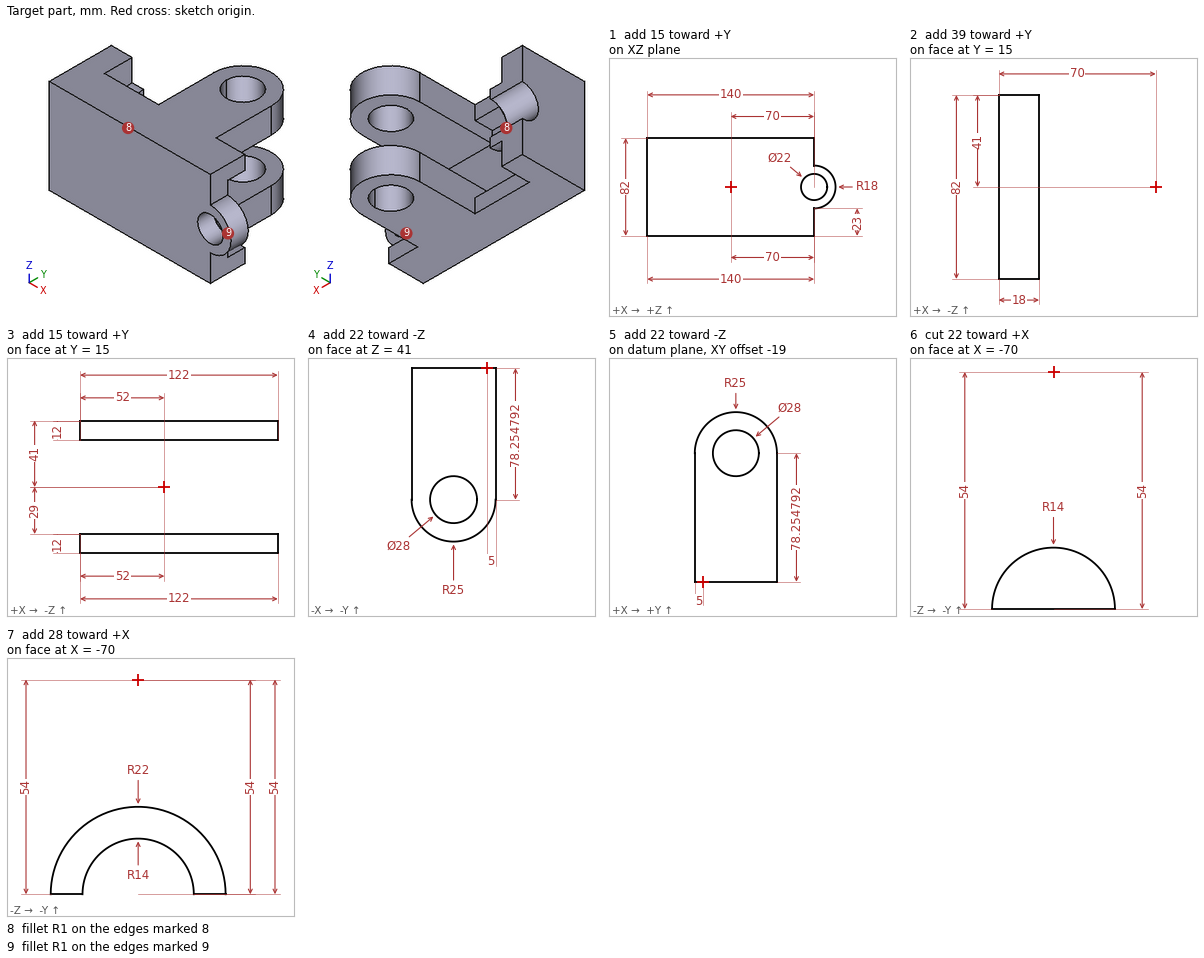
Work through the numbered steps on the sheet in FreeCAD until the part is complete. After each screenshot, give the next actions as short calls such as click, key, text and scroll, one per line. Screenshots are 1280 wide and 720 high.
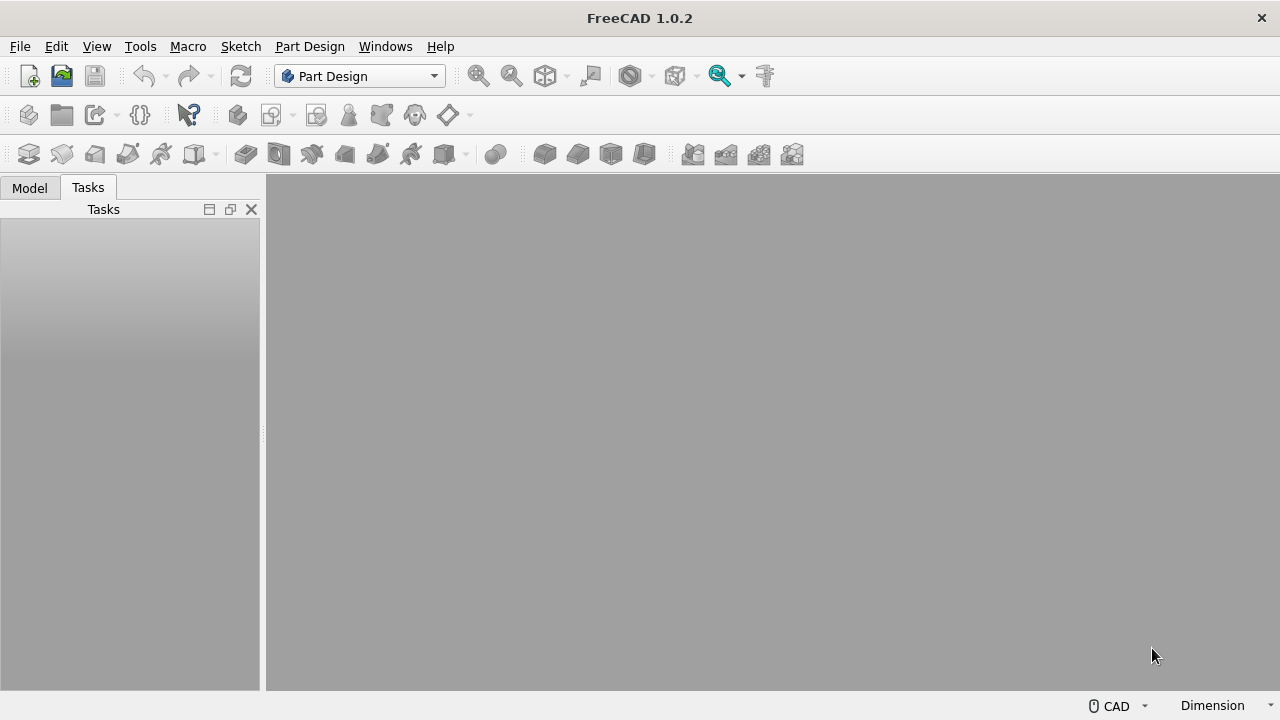
click(29, 76)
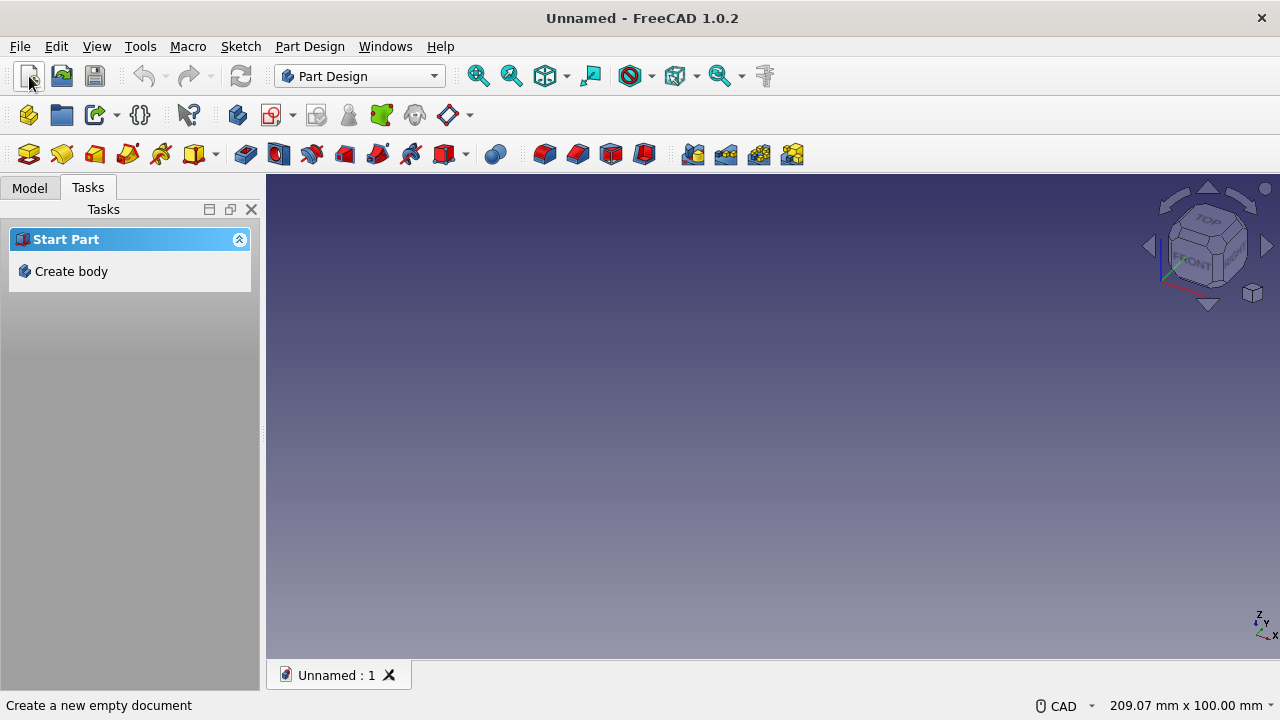
click(270, 116)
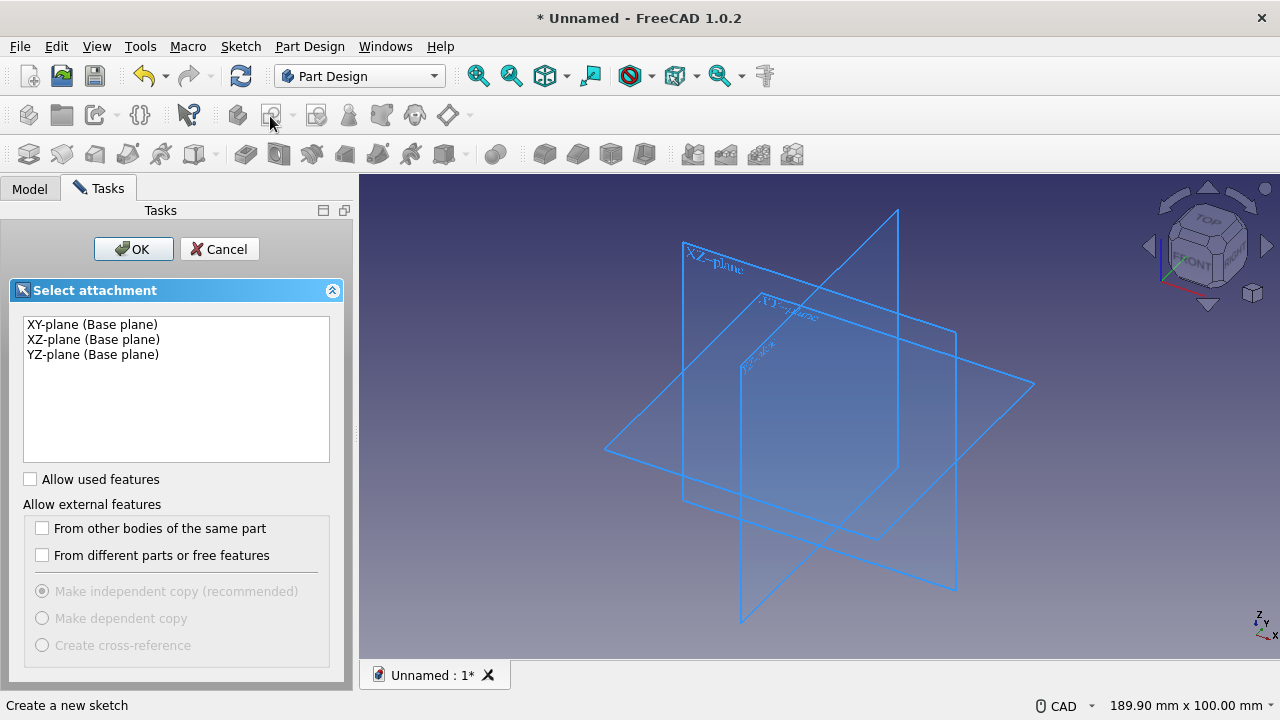
click(84, 340)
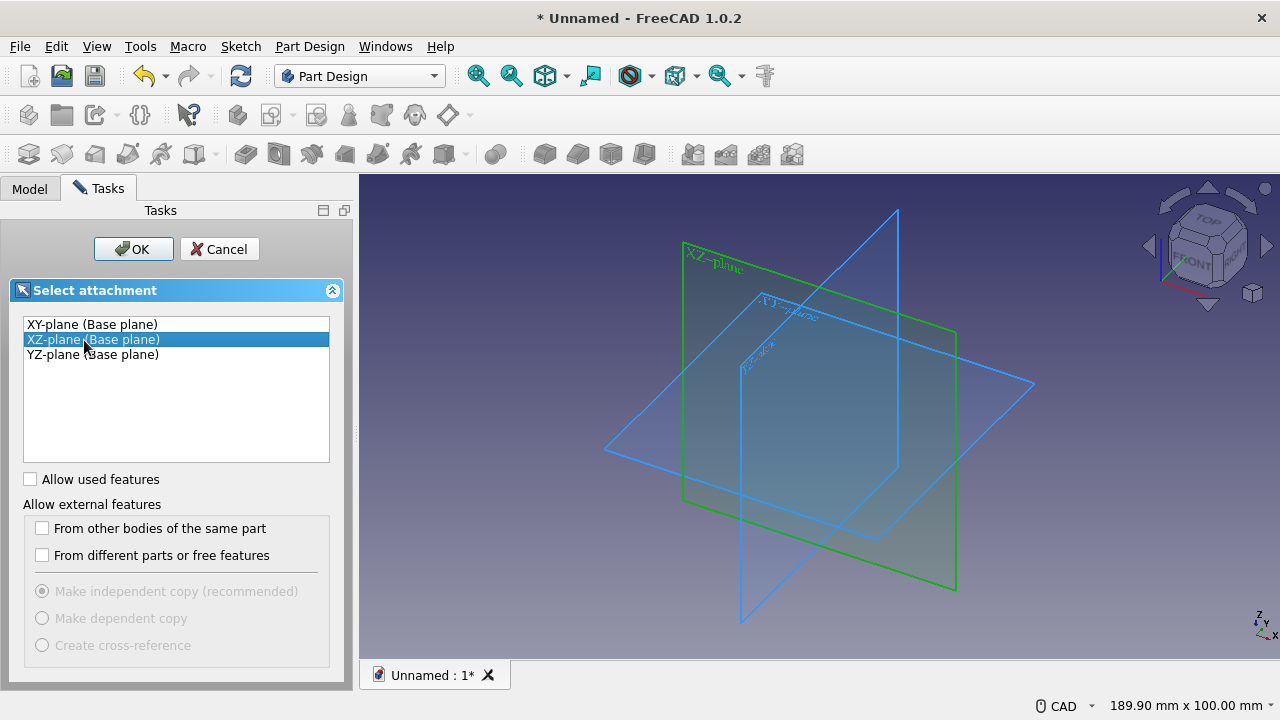
click(134, 249)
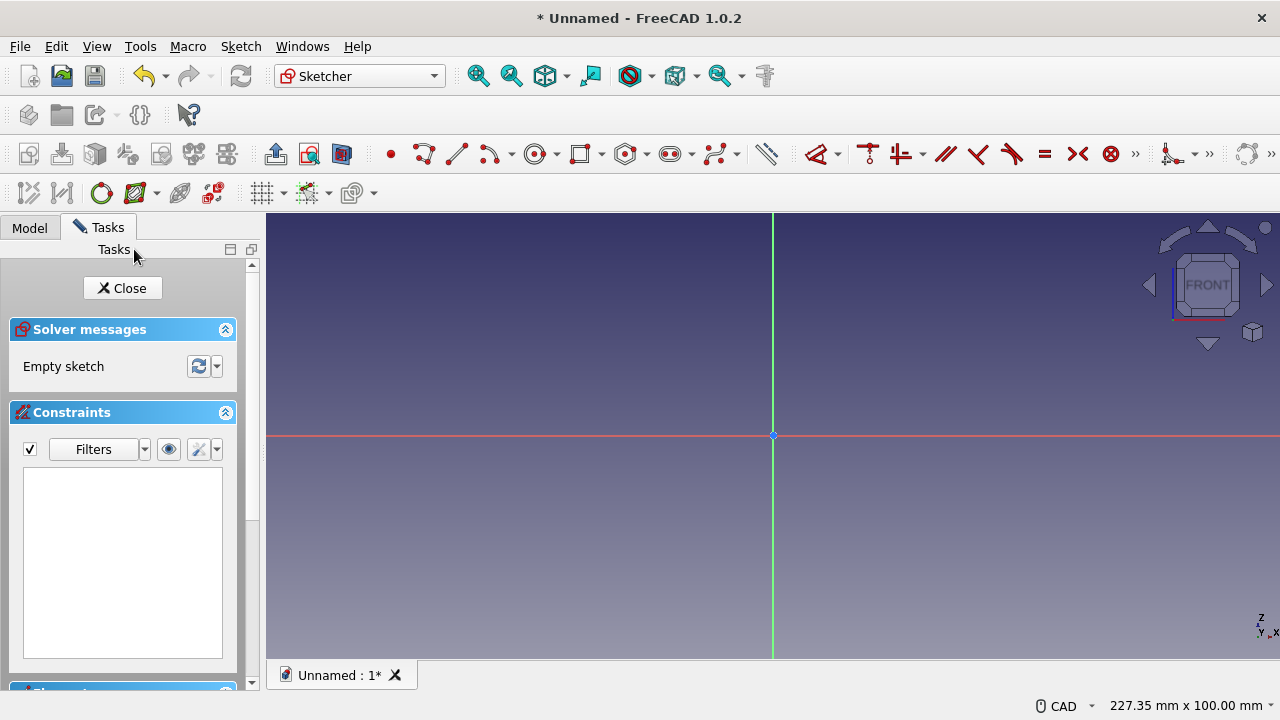
scroll(294, 436, down, 1)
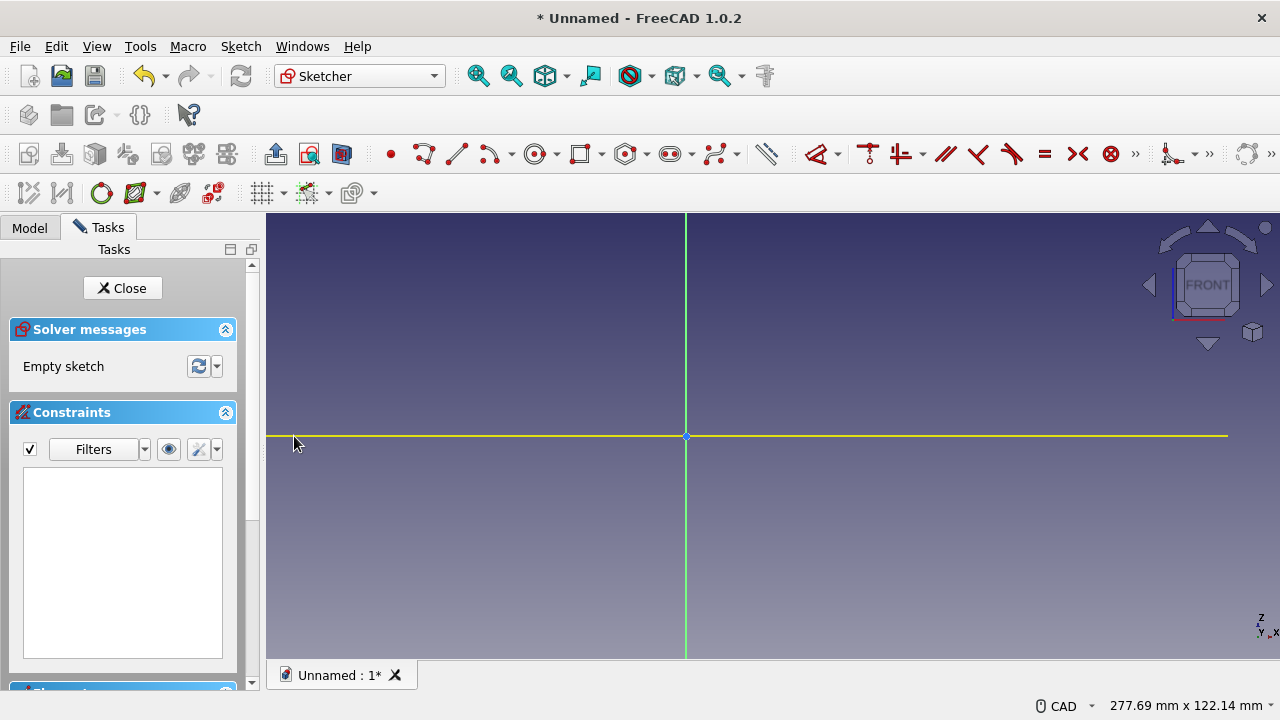
click(424, 154)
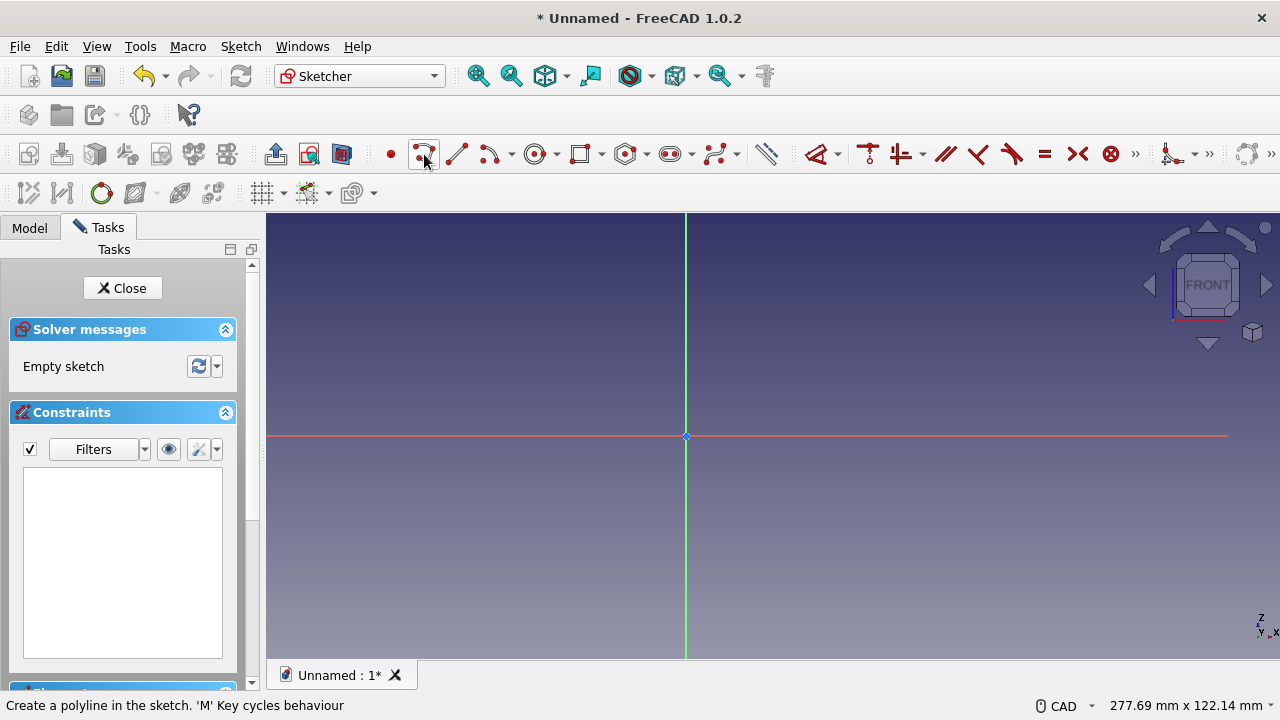
click(942, 502)
click(942, 586)
click(431, 586)
click(431, 286)
click(942, 286)
click(942, 370)
right_click(942, 370)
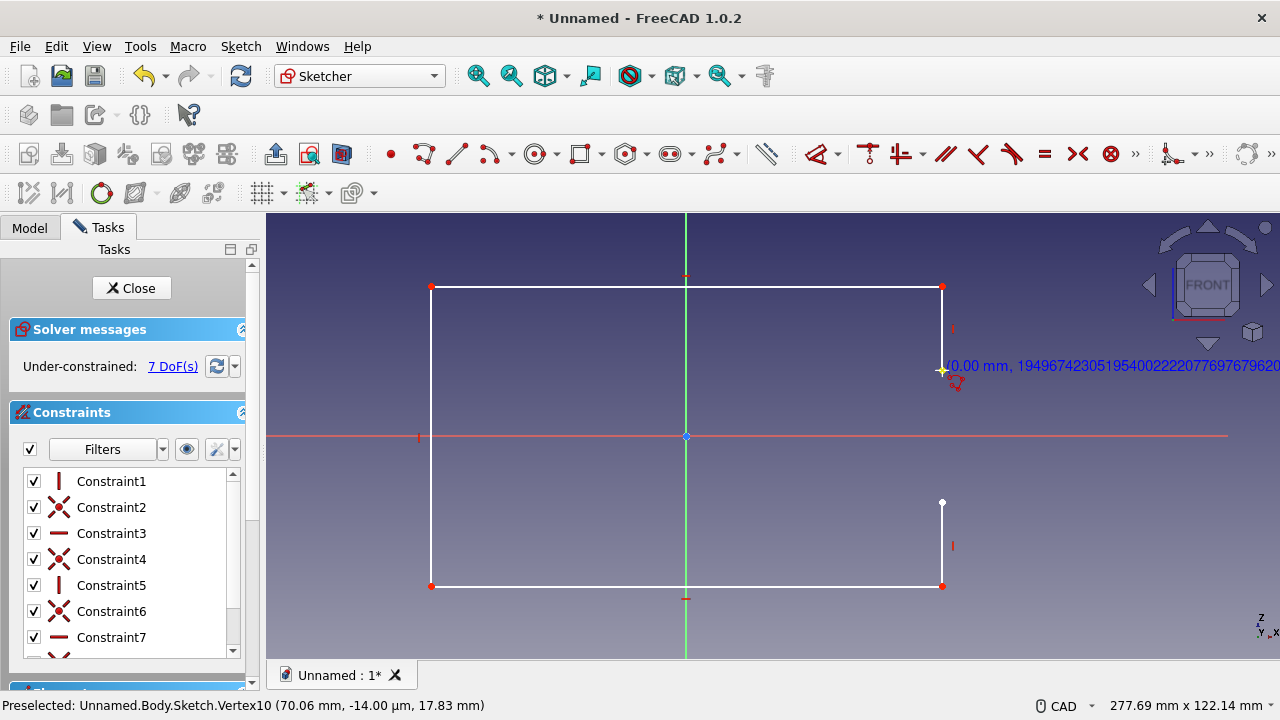
key(g)
key(3)
key(a)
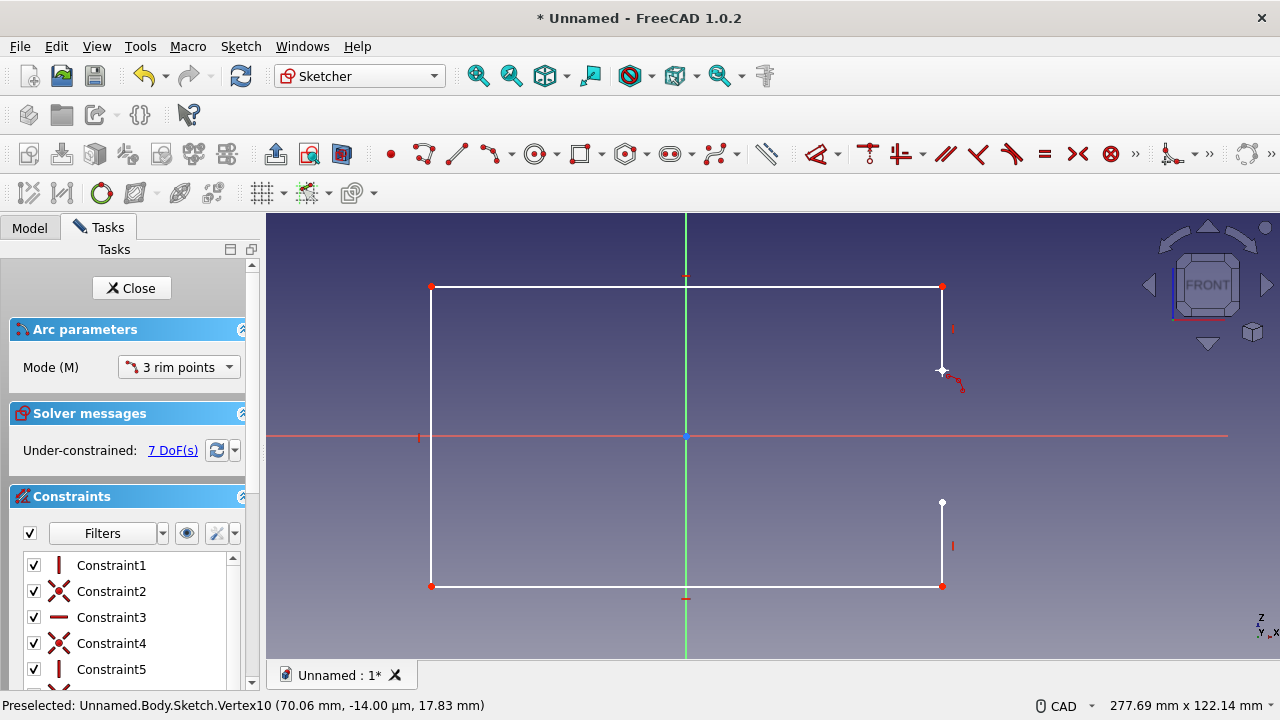
click(942, 371)
click(942, 503)
click(1004, 456)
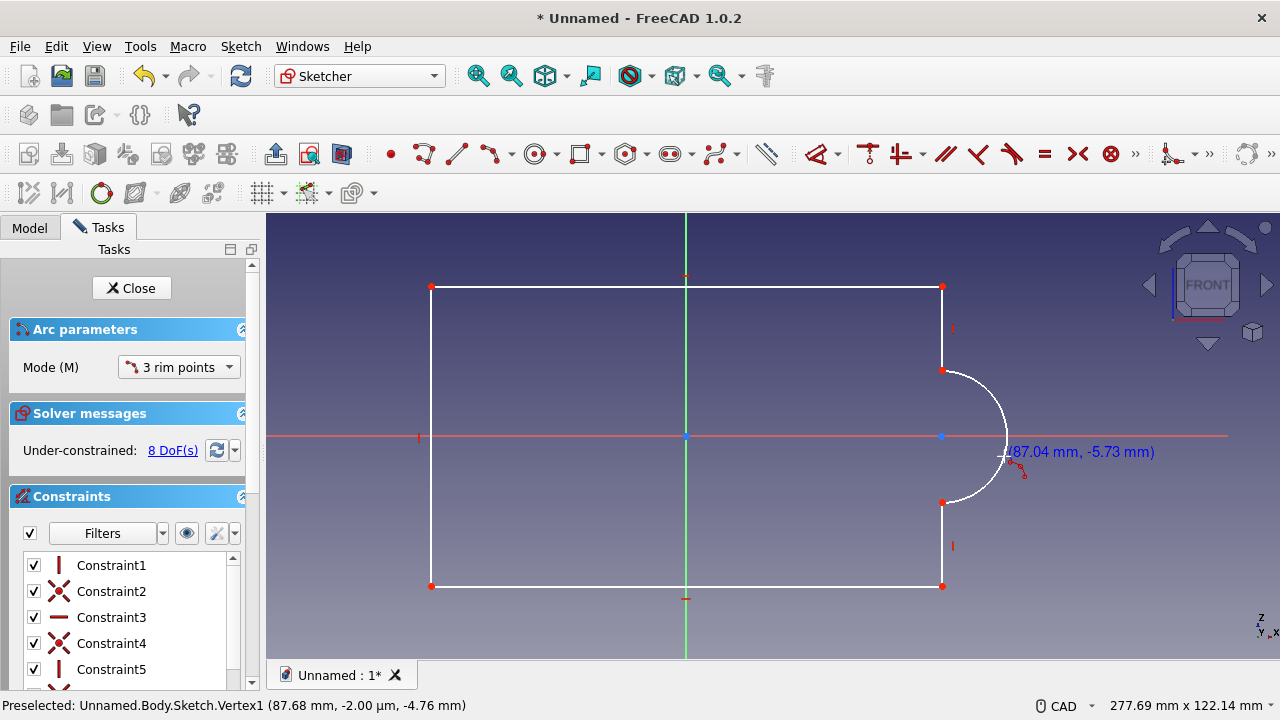
click(534, 154)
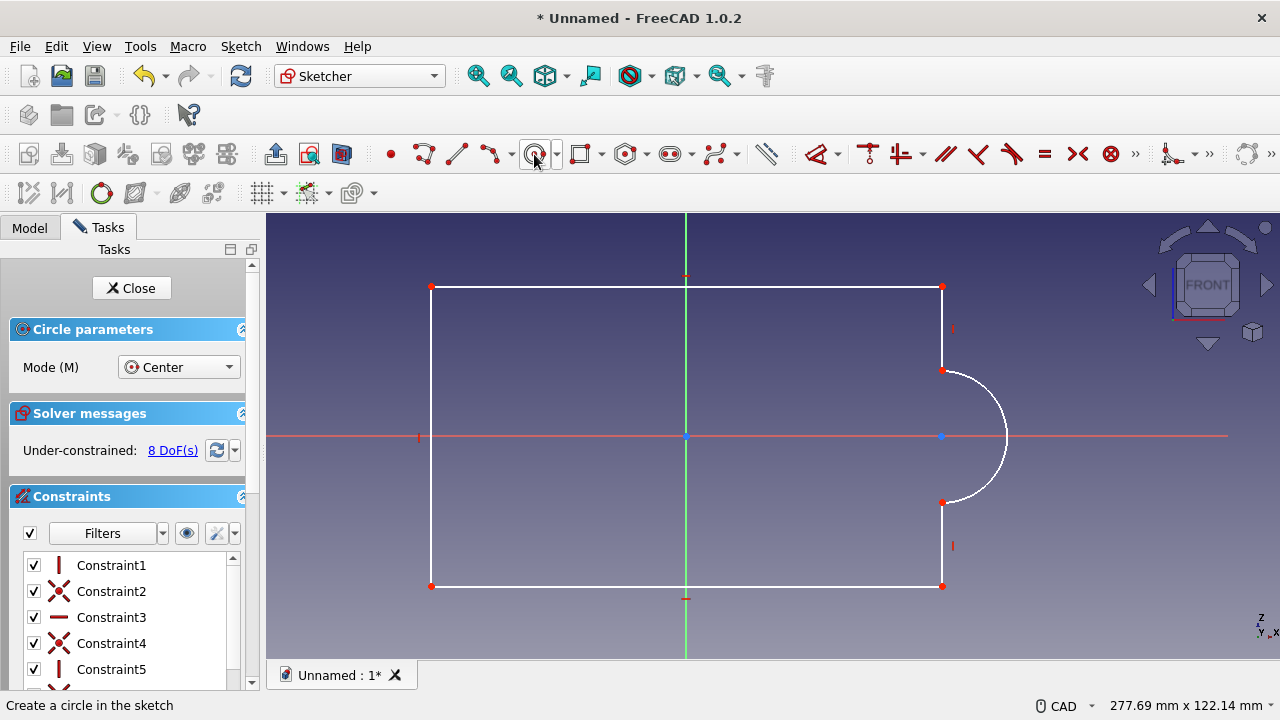
click(942, 436)
click(970, 408)
key(Escape)